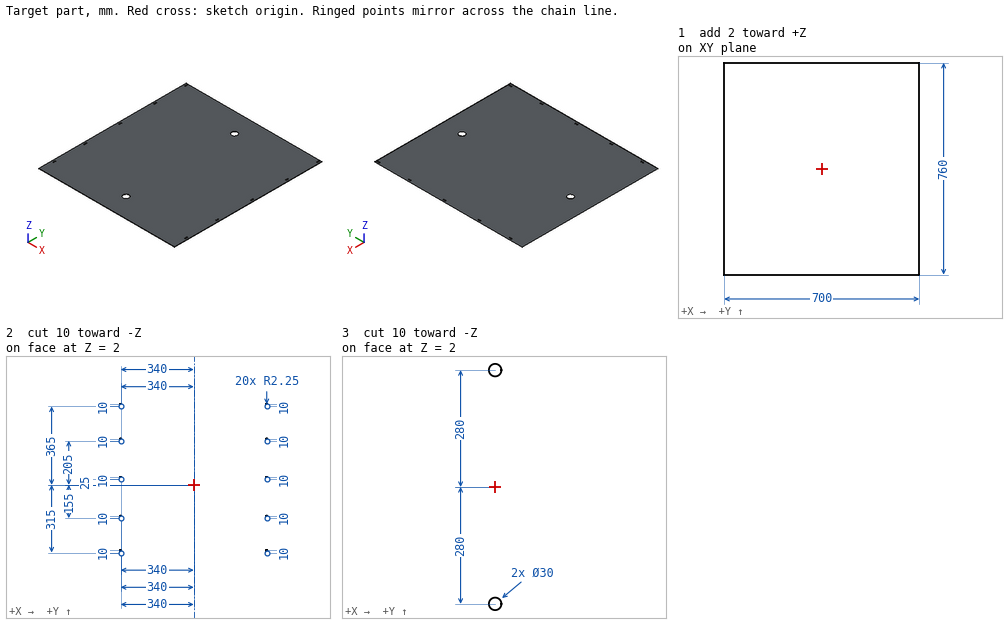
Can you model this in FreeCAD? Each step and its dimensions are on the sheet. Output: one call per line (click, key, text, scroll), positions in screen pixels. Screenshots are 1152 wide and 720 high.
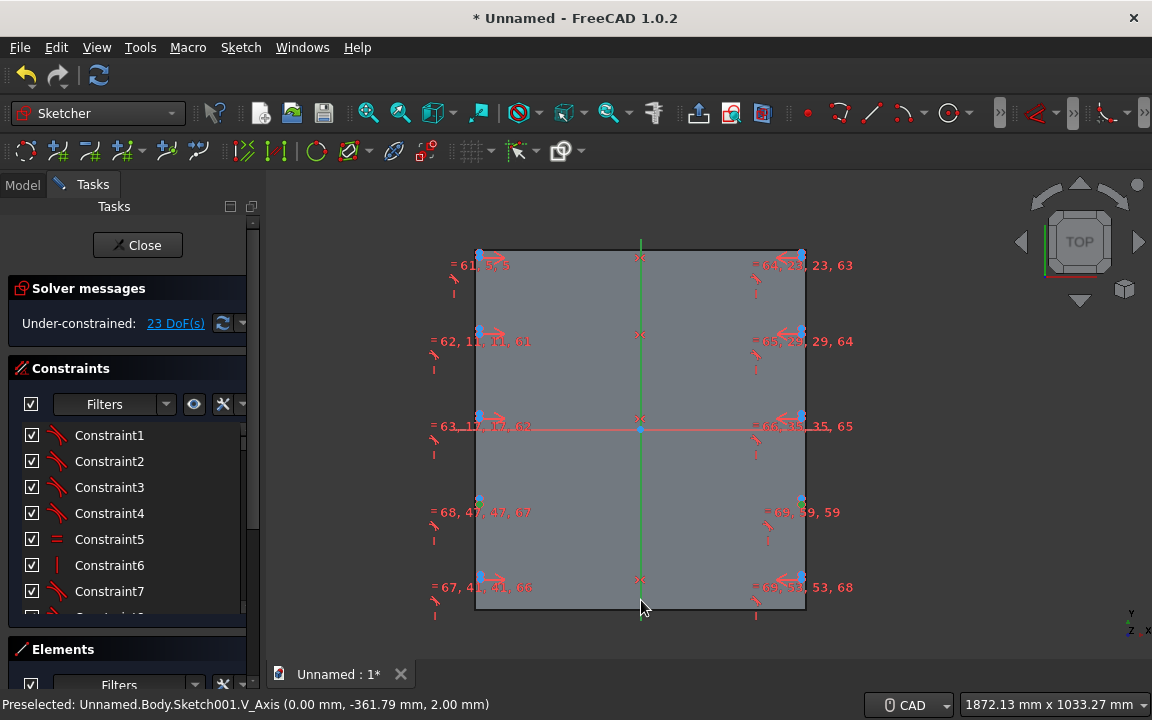
key(s)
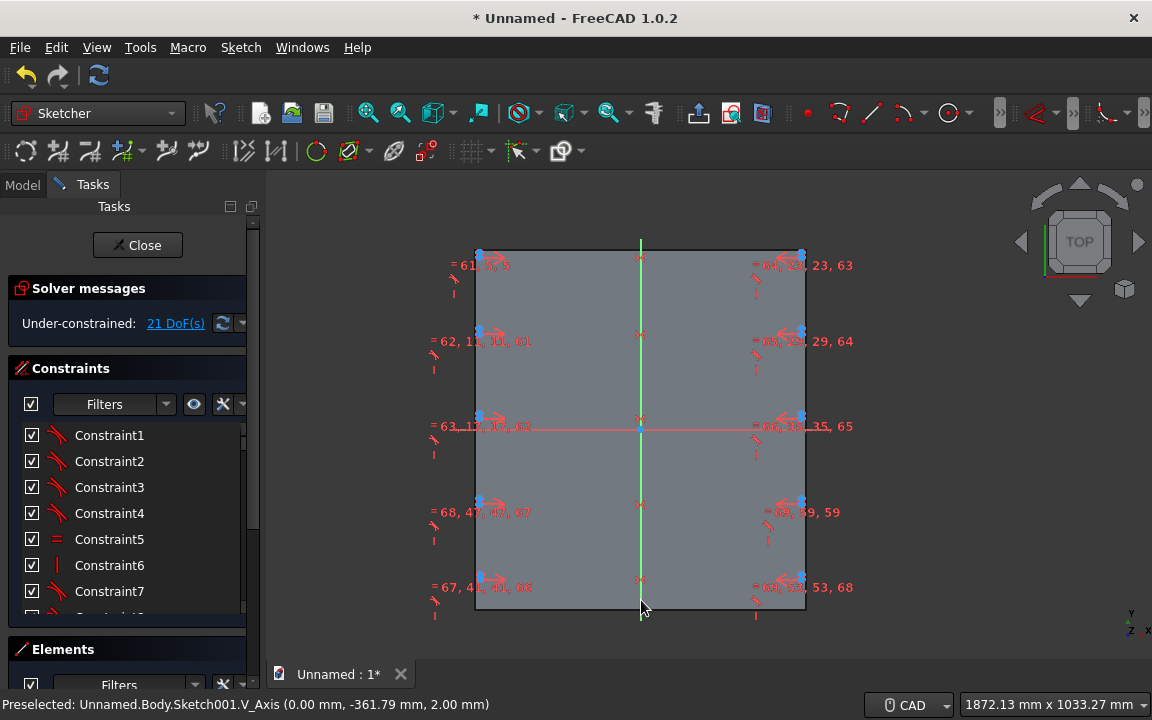
scroll(480, 259, up, 19)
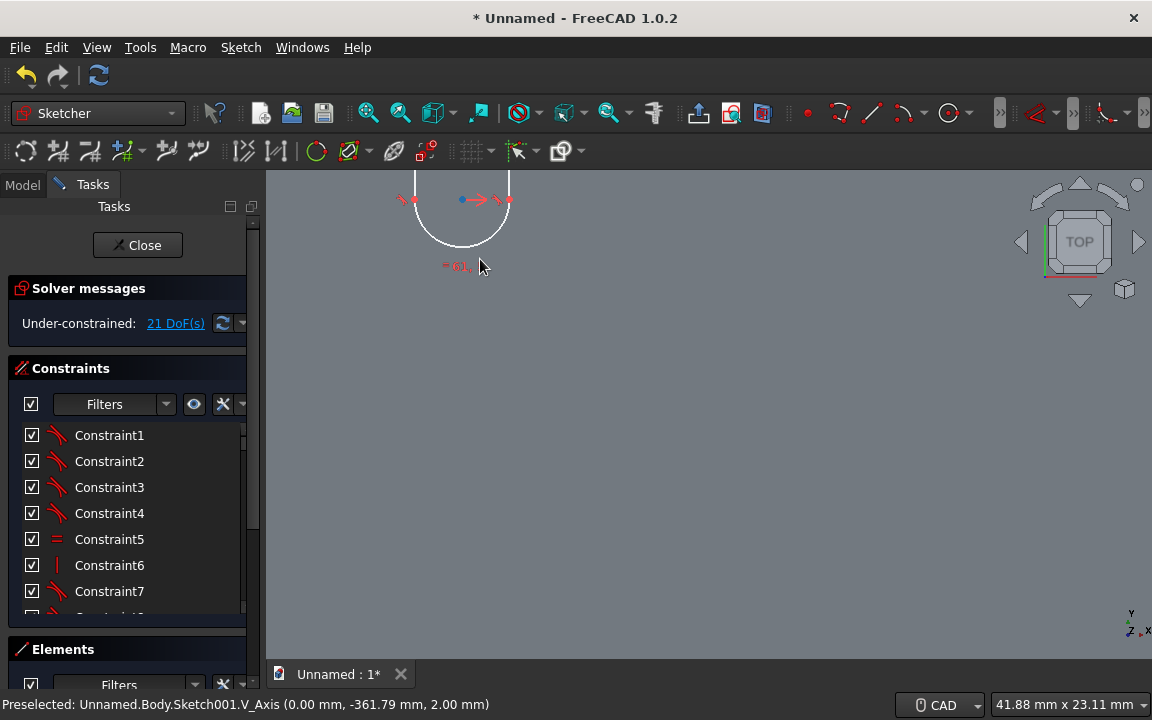
click(462, 247)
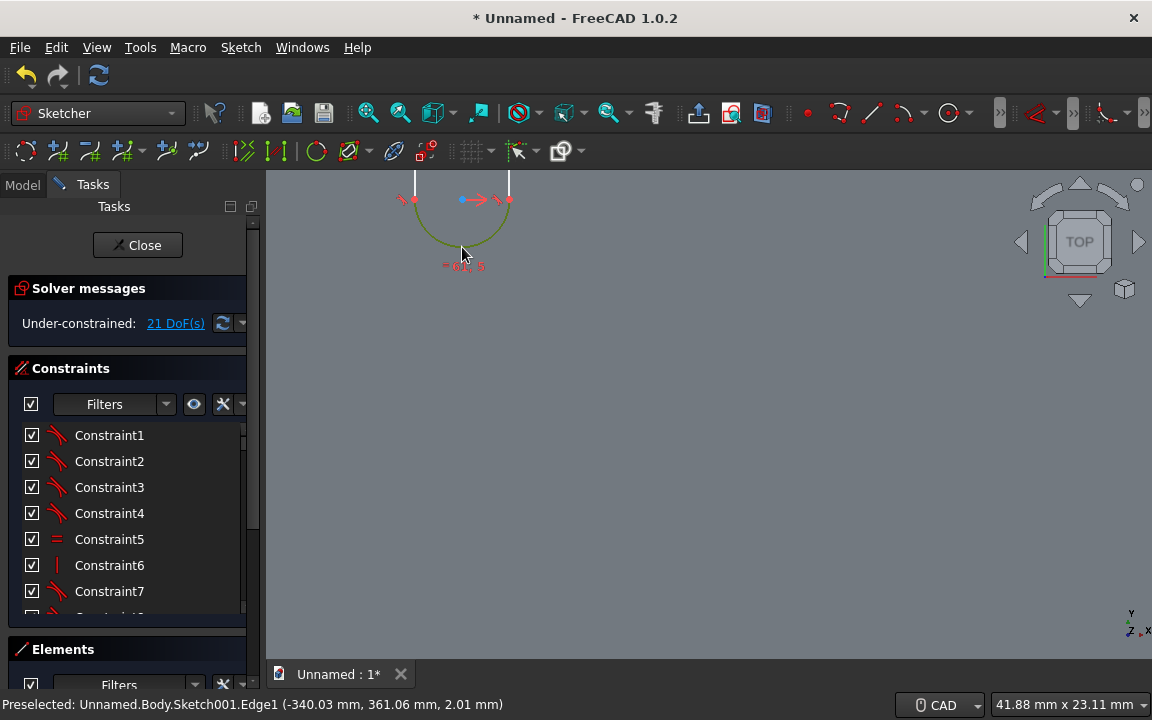
click(1058, 114)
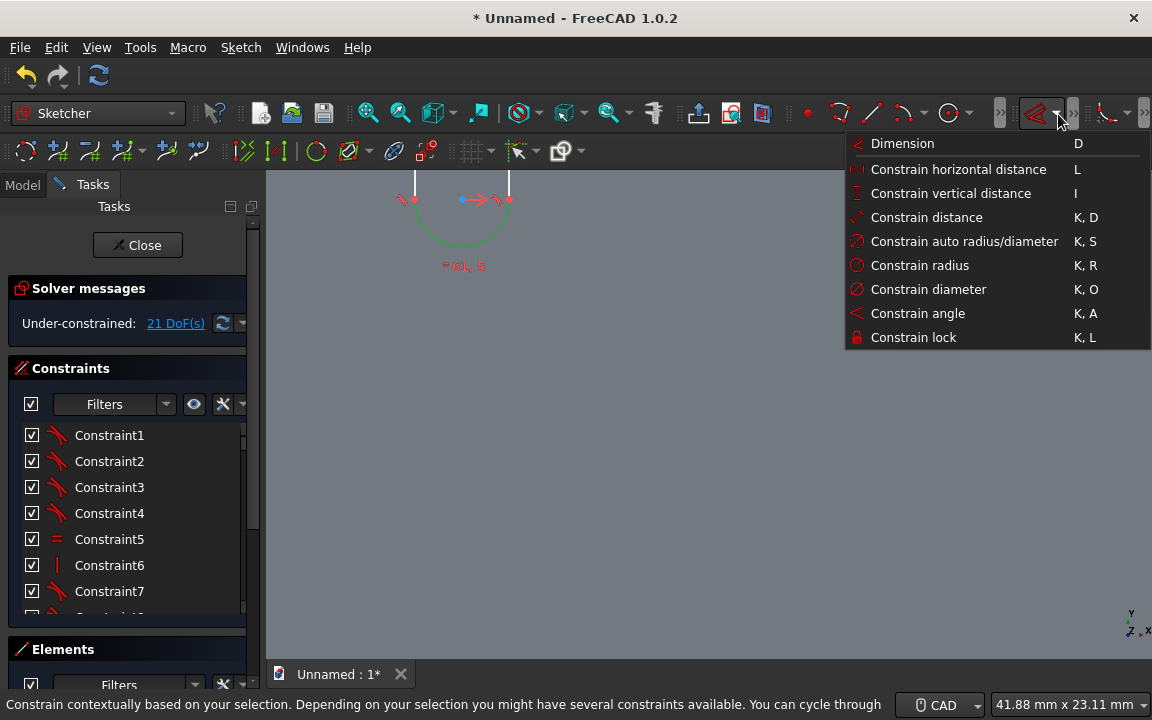
click(998, 265)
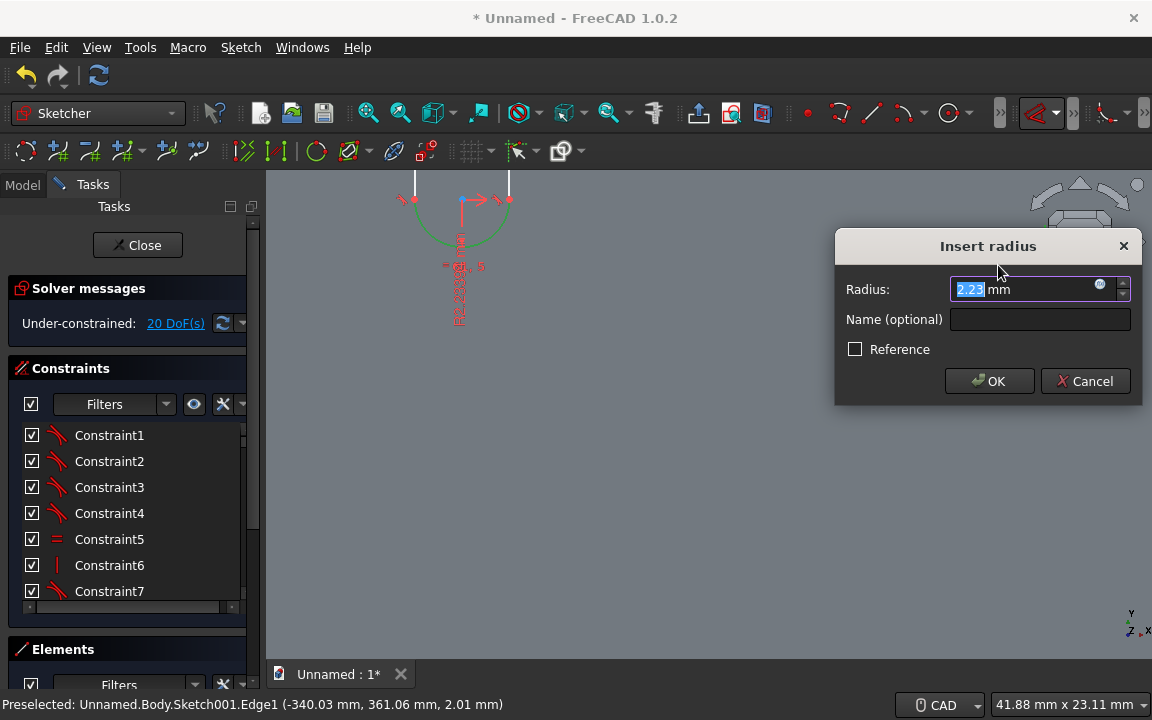
text(2.25)
key(Return)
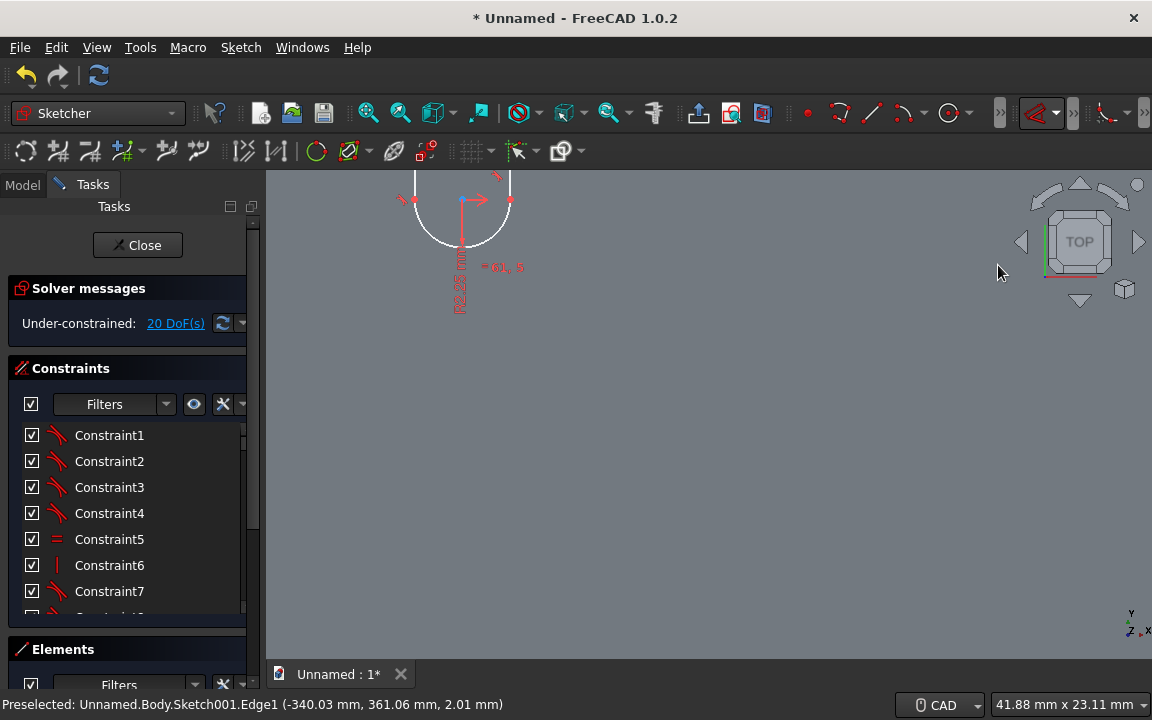
scroll(640, 414, down, 15)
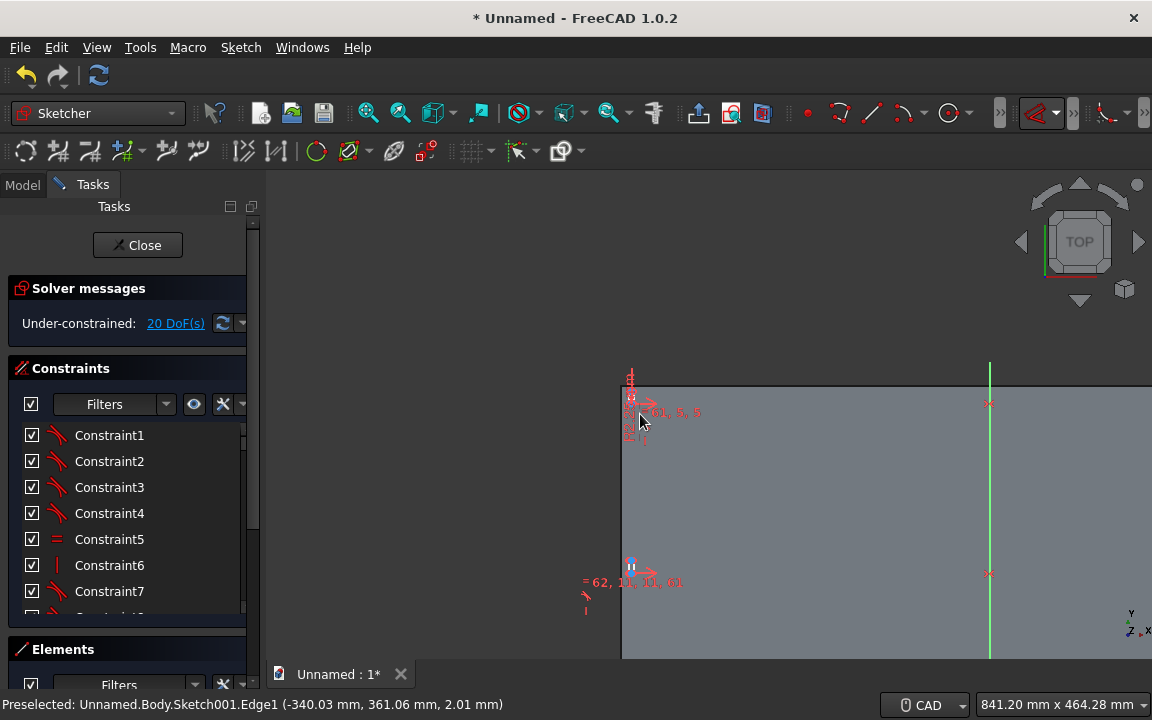
scroll(437, 216, down, 5)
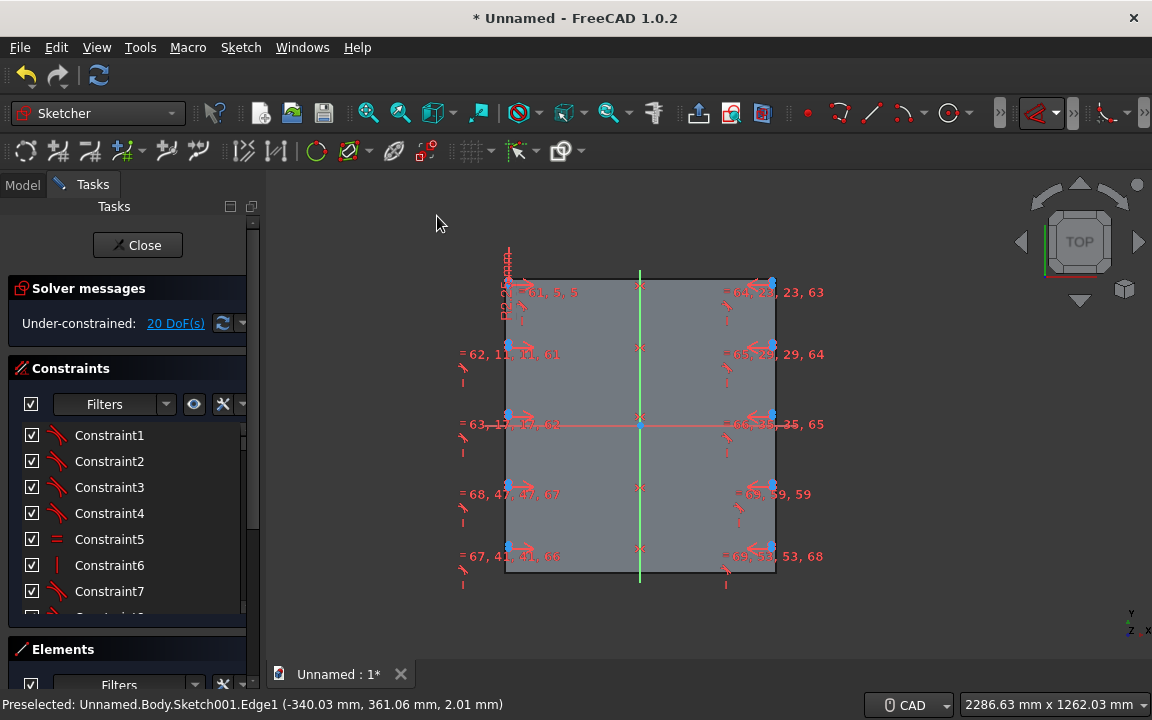
scroll(508, 284, up, 12)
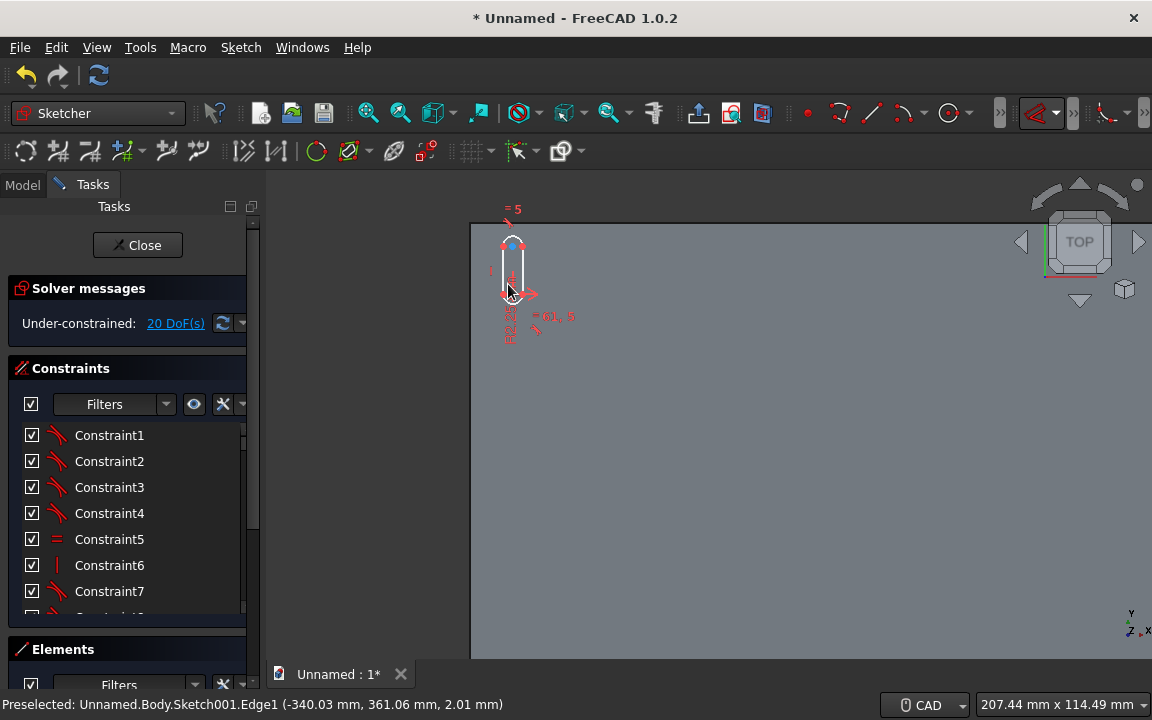
click(503, 280)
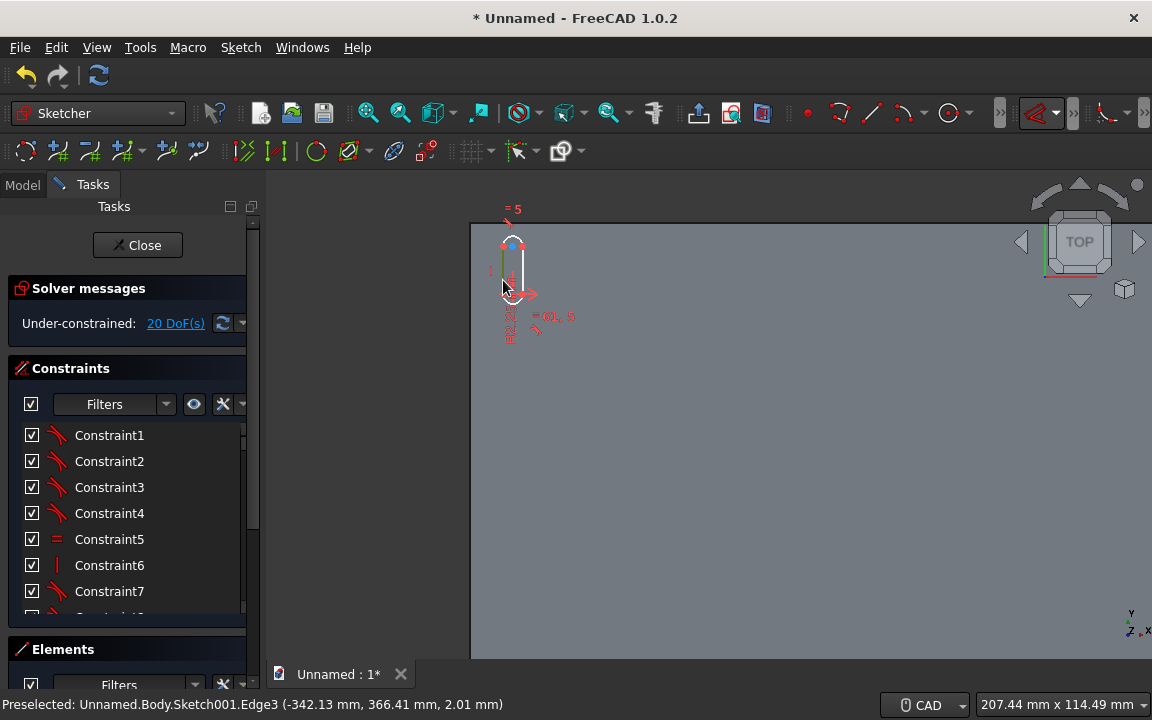
click(1058, 114)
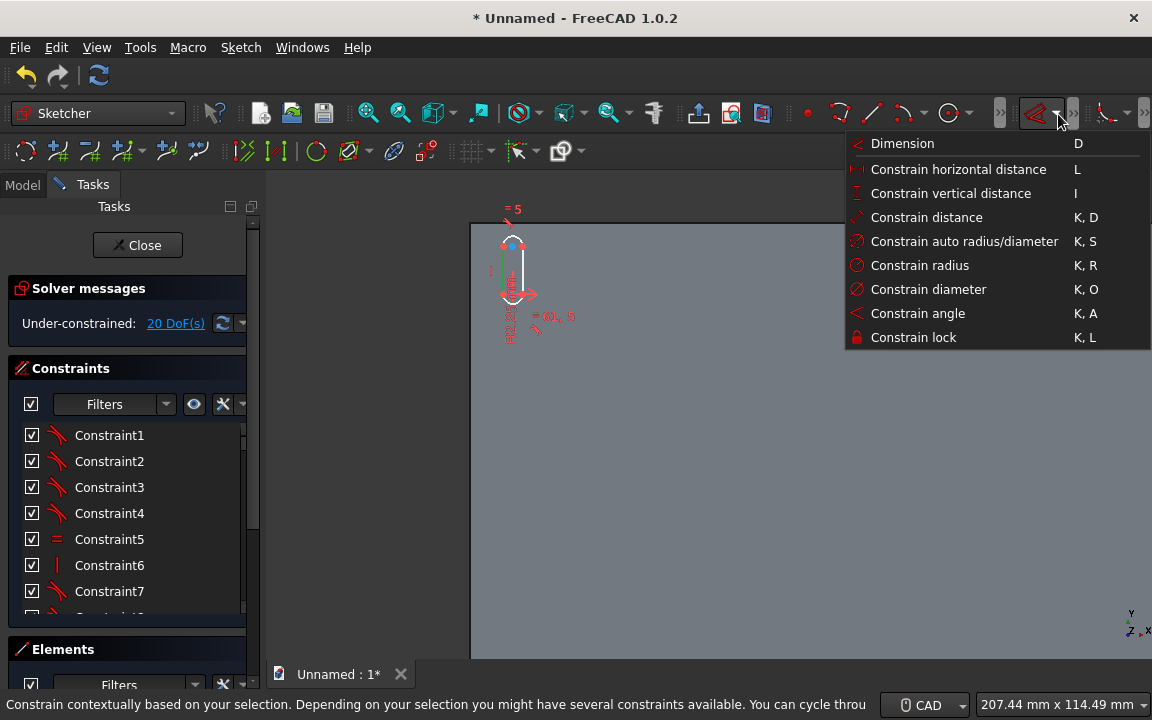
click(998, 193)